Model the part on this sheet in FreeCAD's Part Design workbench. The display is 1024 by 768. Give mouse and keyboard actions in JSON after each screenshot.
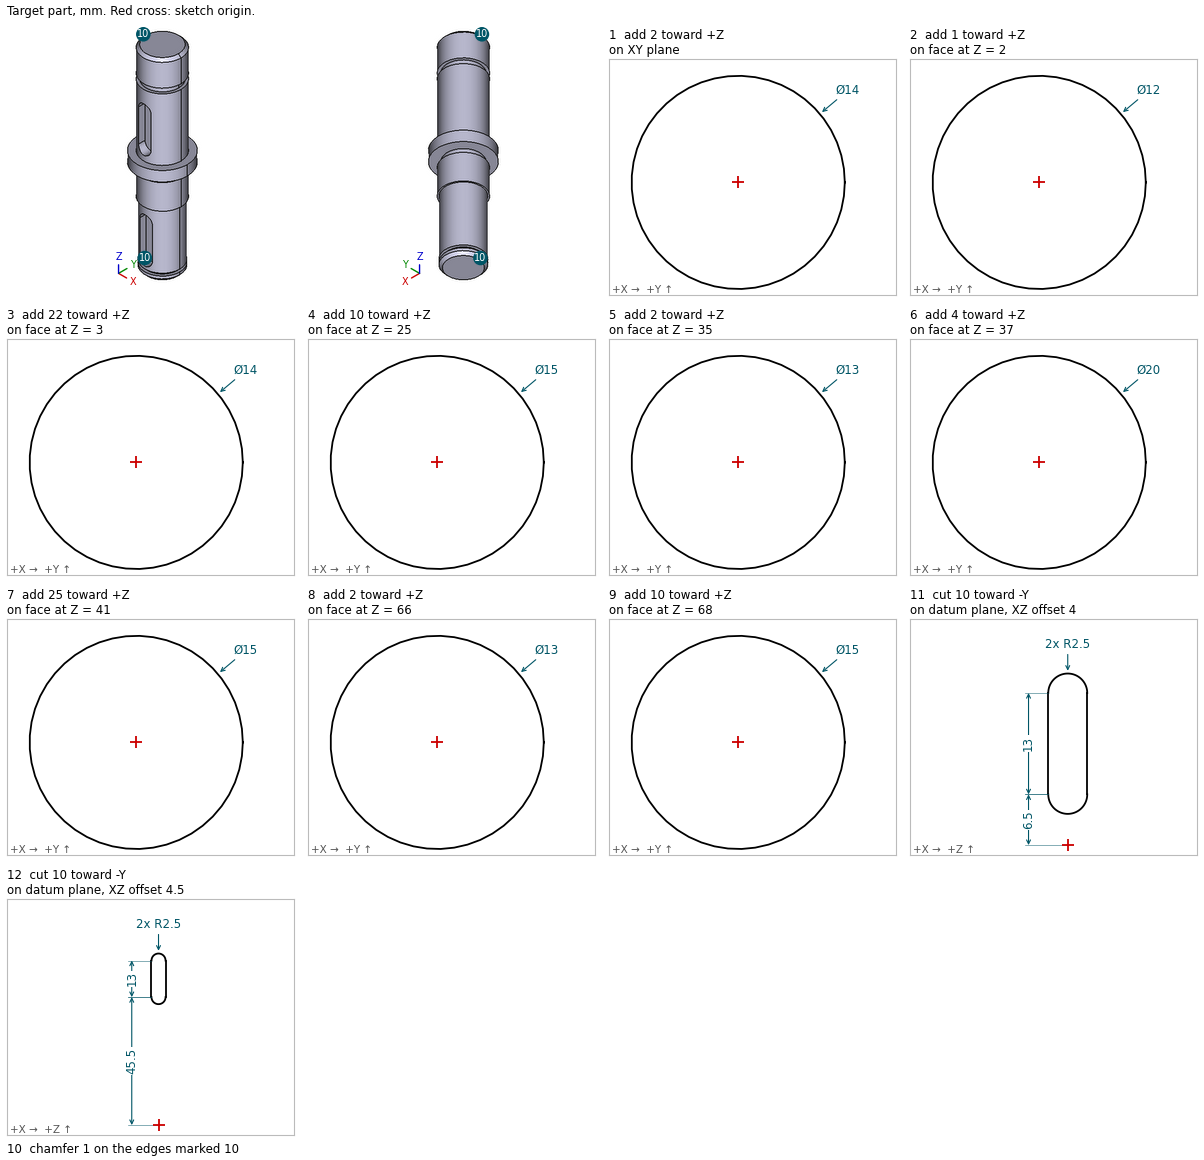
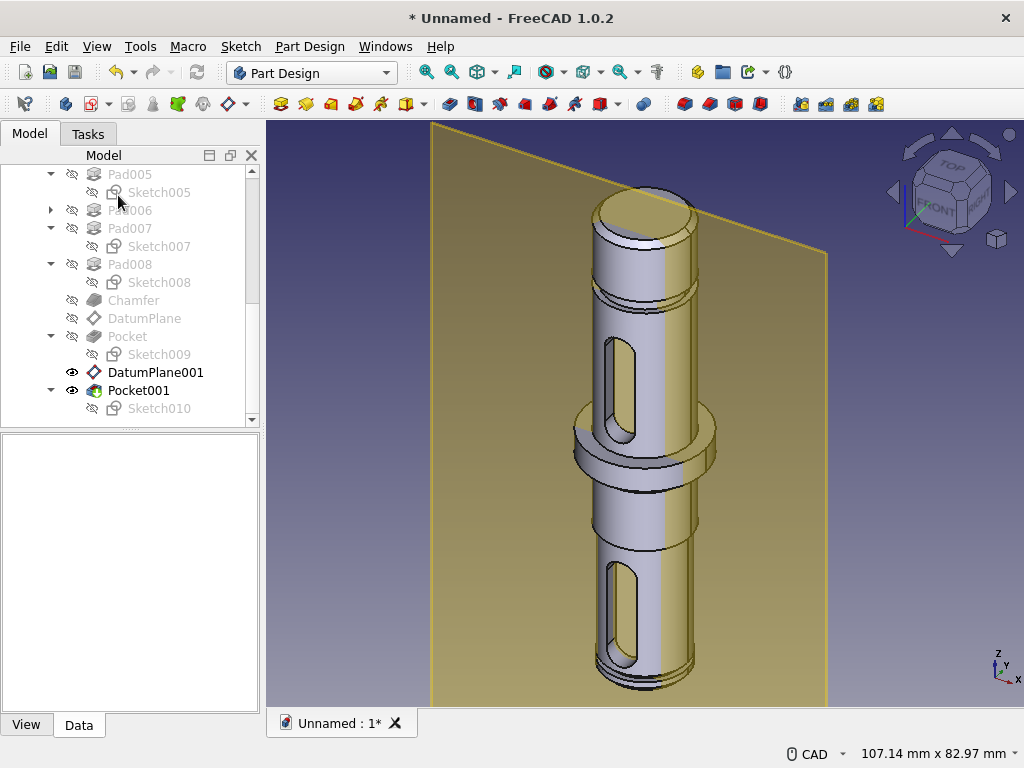
{"action": "left_click", "coordinate": [117, 372]}
{"action": "key", "text": "space"}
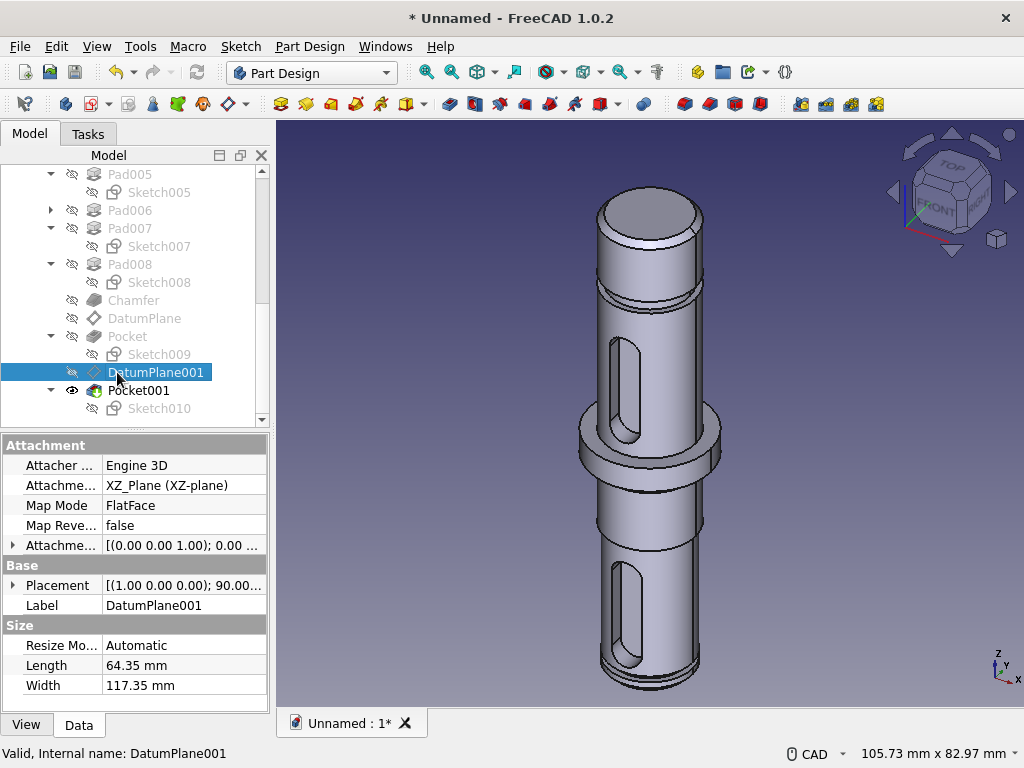
{"action": "key", "text": "0"}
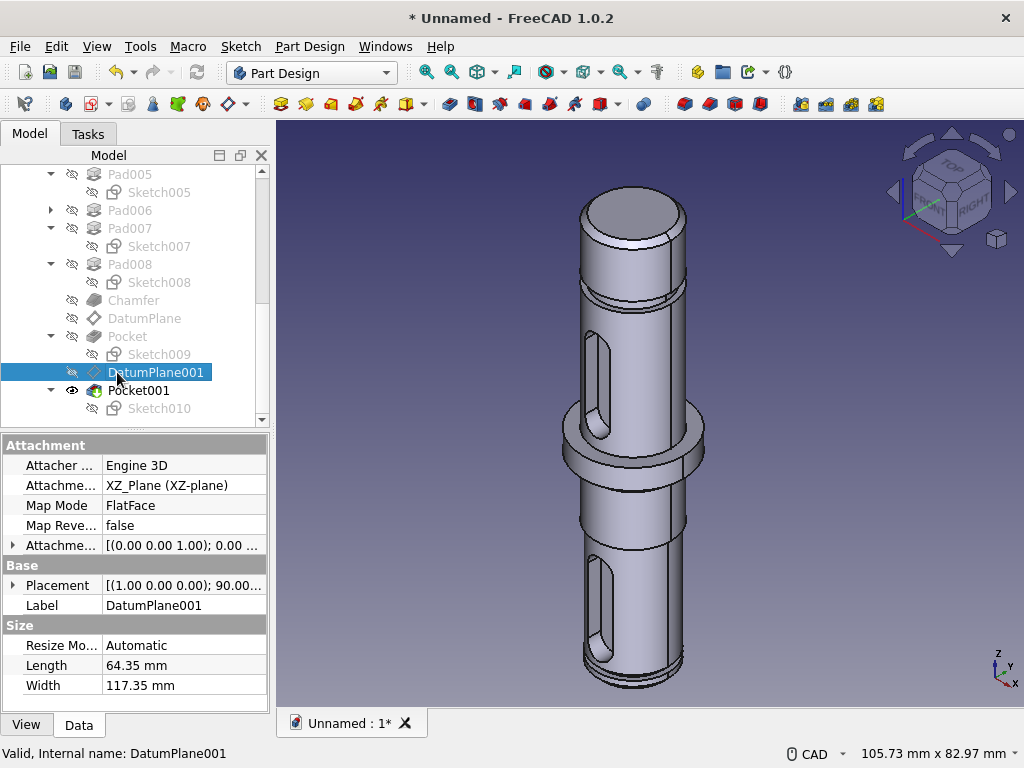
{"action": "left_click", "coordinate": [427, 72]}